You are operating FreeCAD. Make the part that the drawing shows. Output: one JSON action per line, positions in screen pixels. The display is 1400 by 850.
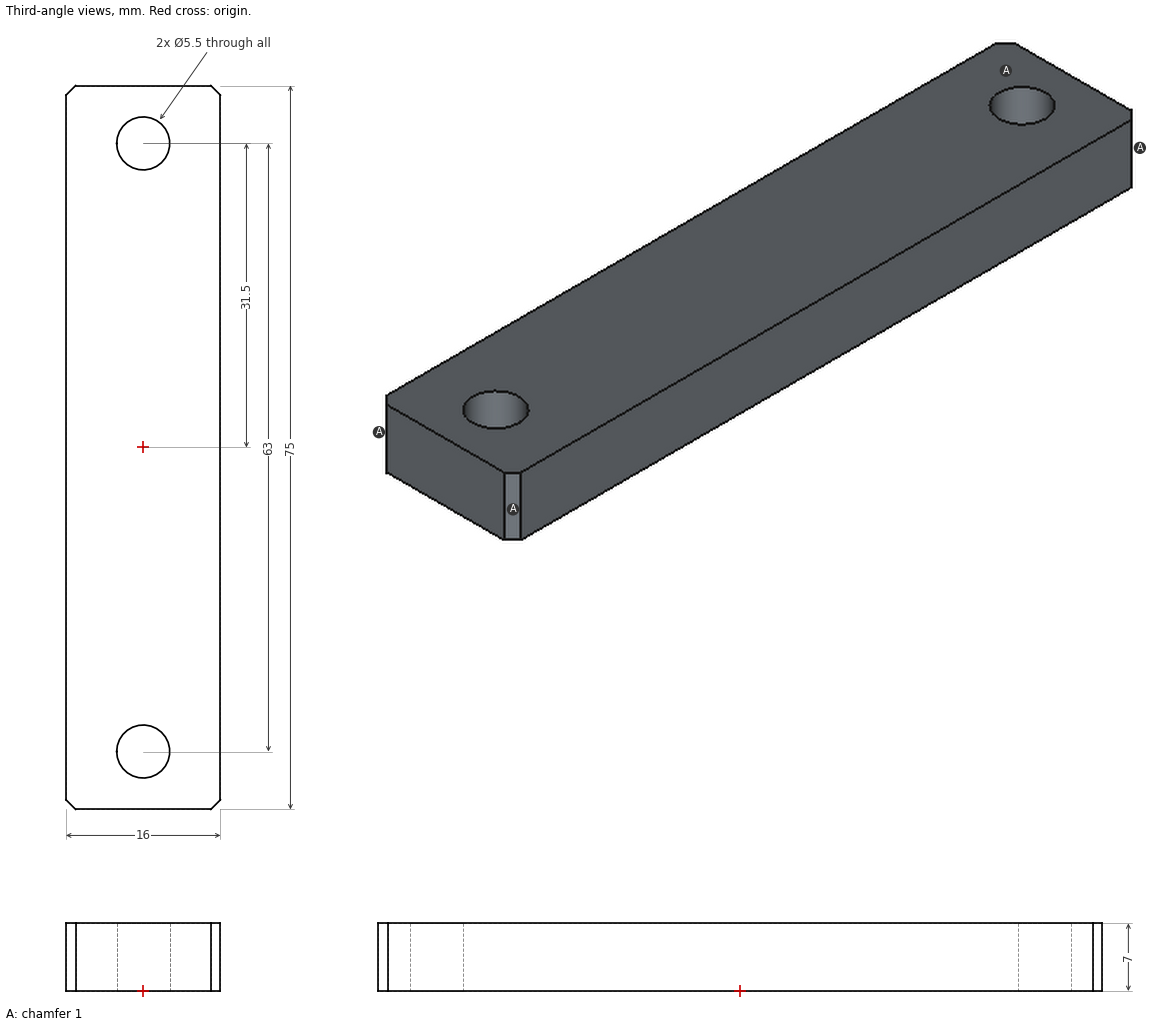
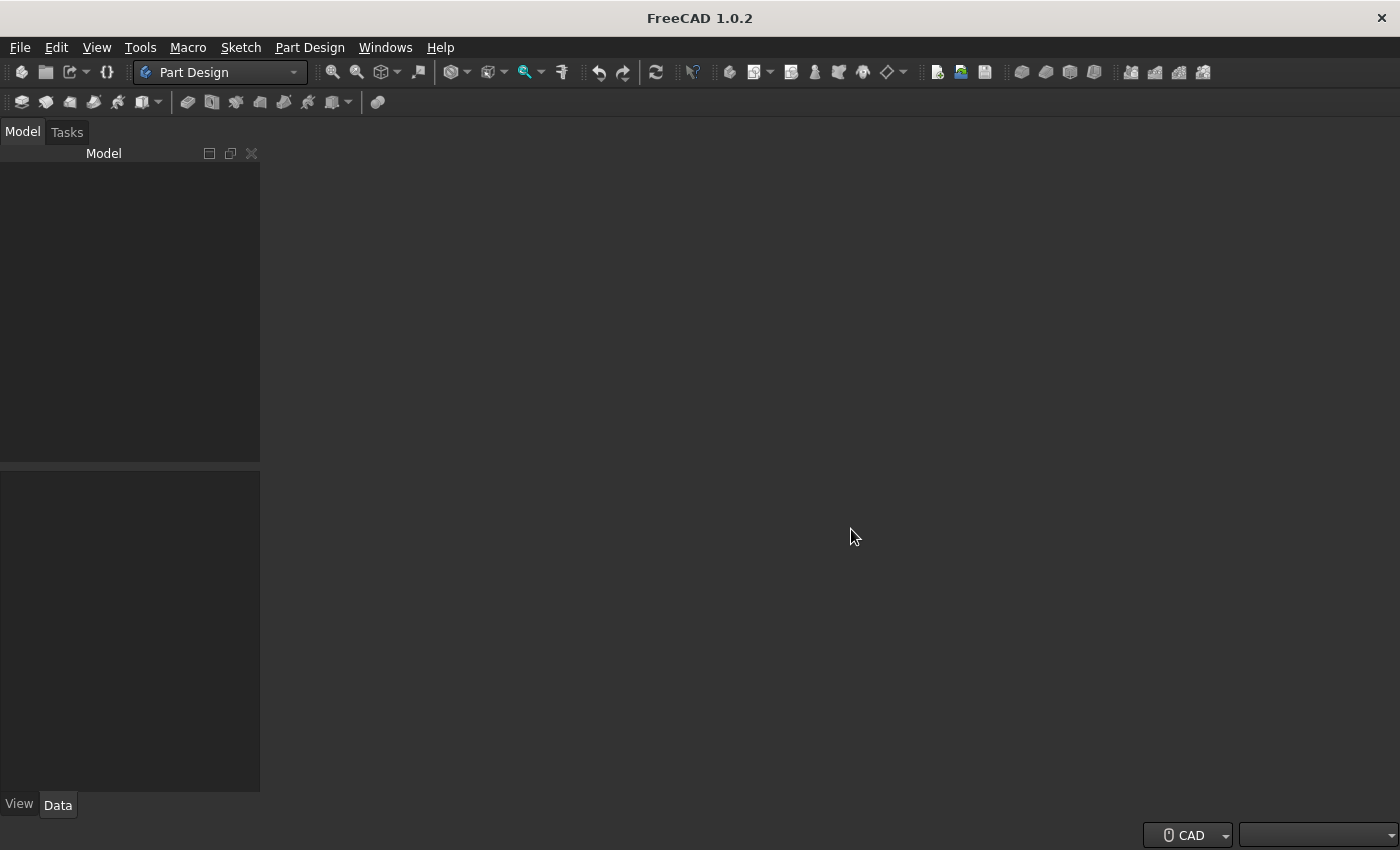
{"action": "left_click", "coordinate": [938, 72]}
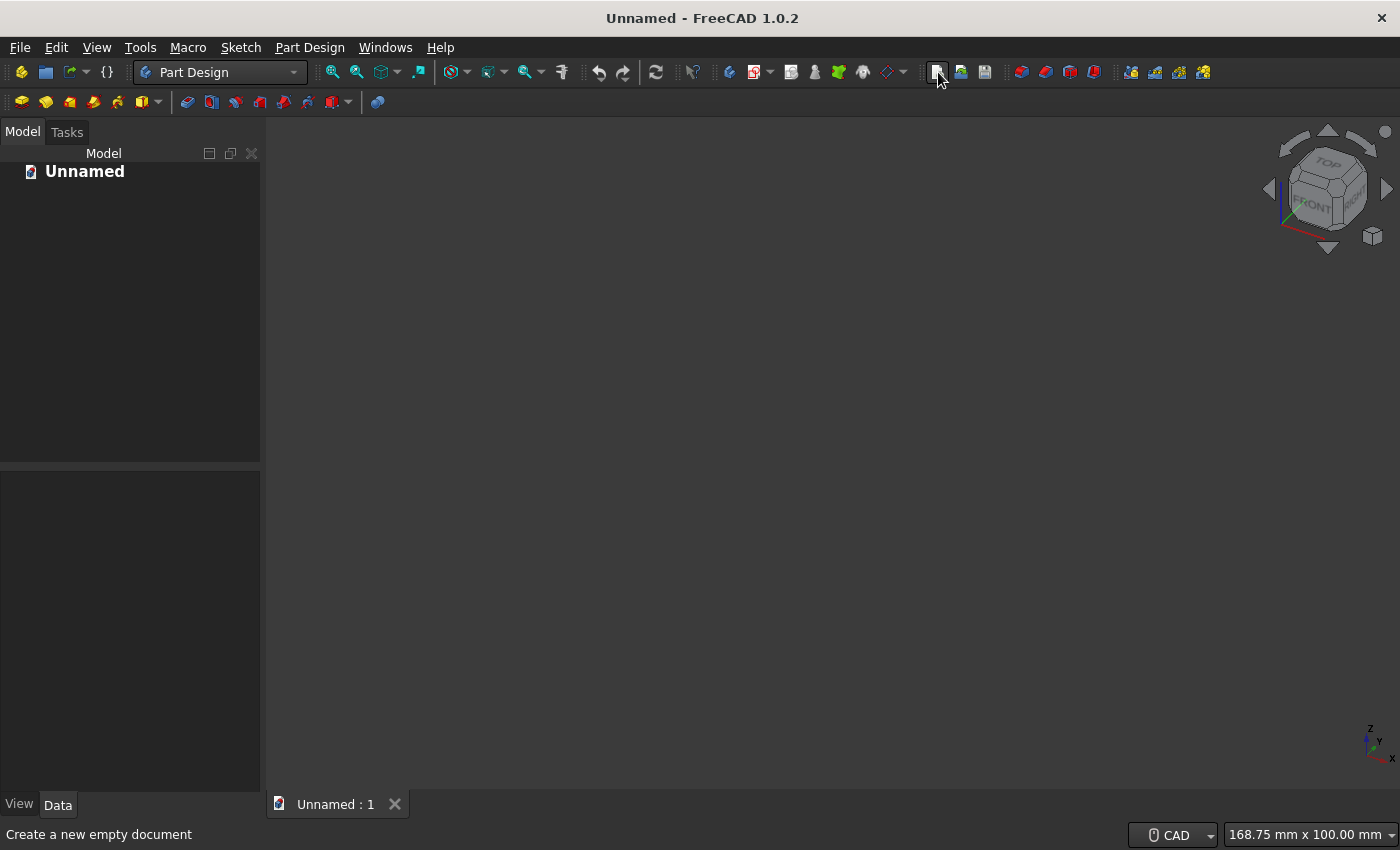
{"action": "left_click", "coordinate": [754, 72]}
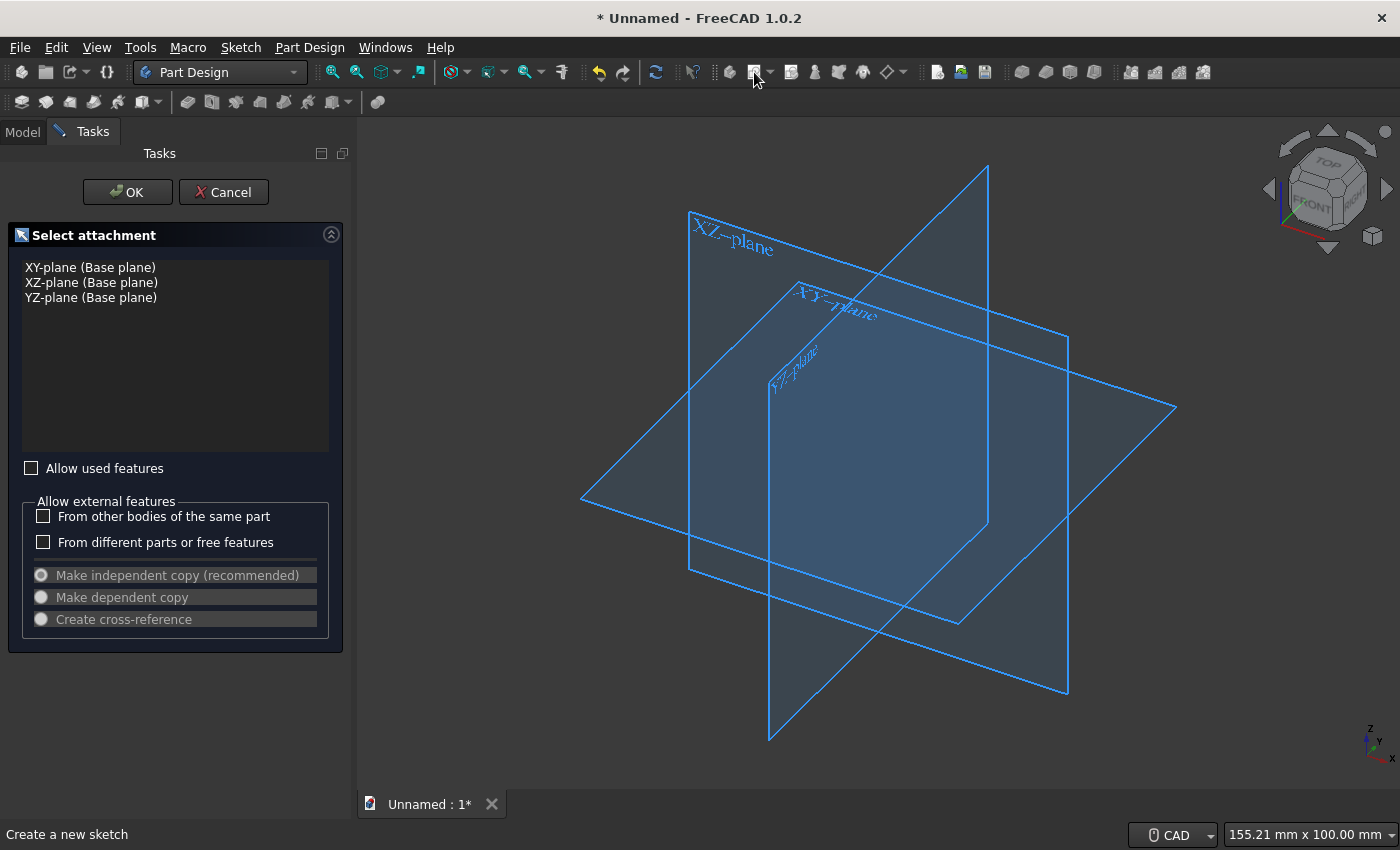
{"action": "left_click", "coordinate": [82, 268]}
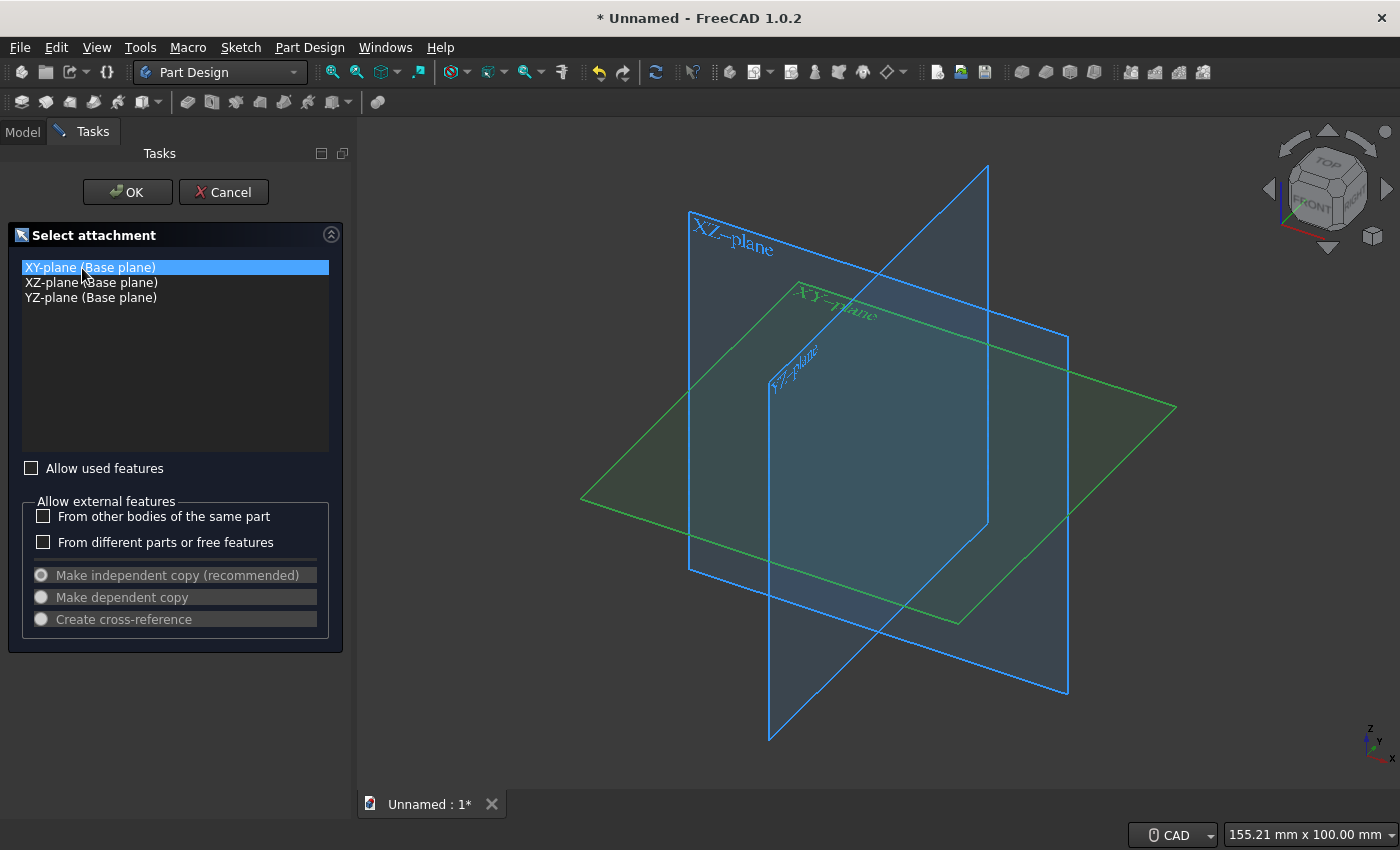
{"action": "left_click", "coordinate": [128, 192]}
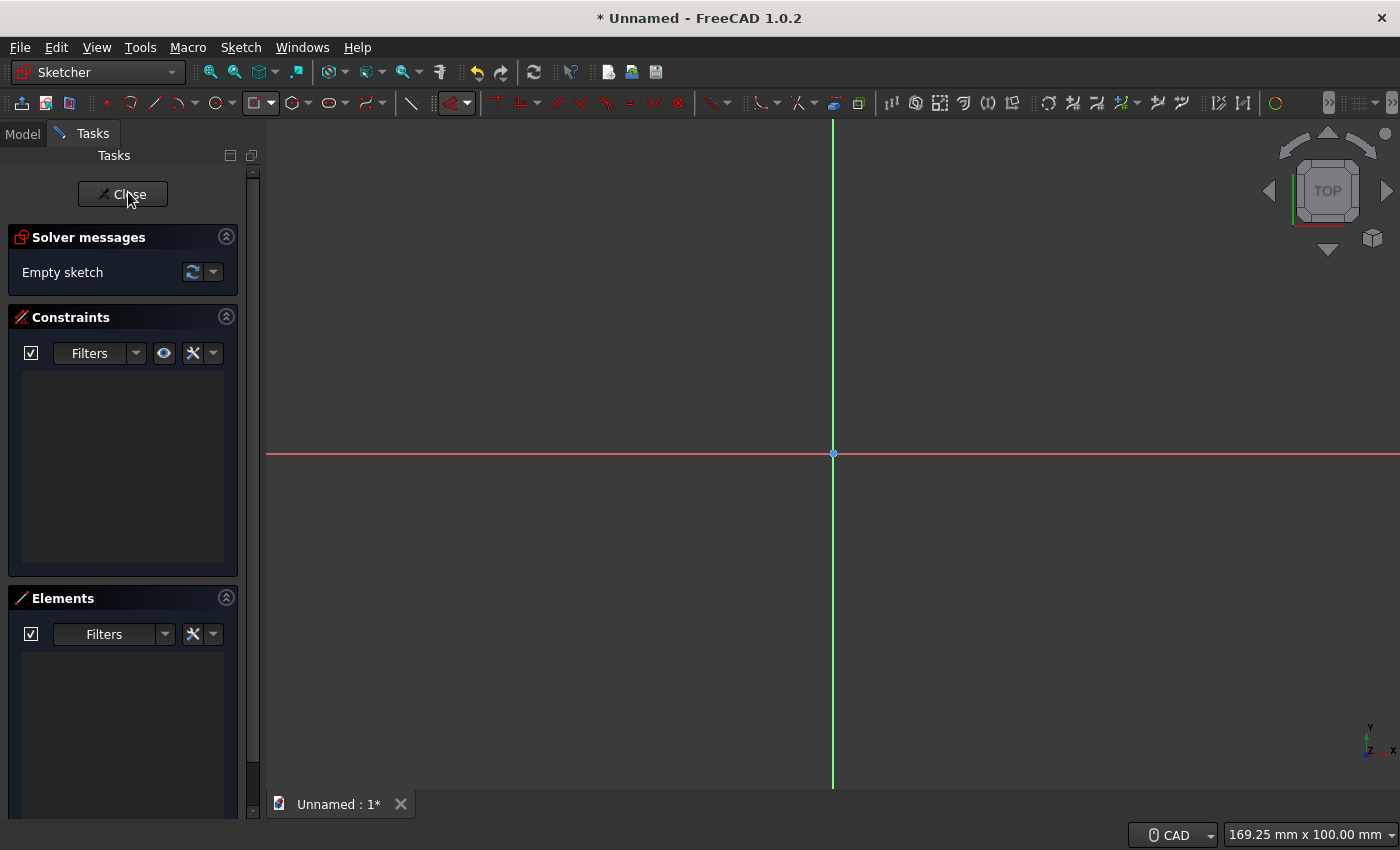
{"action": "left_click", "coordinate": [254, 104]}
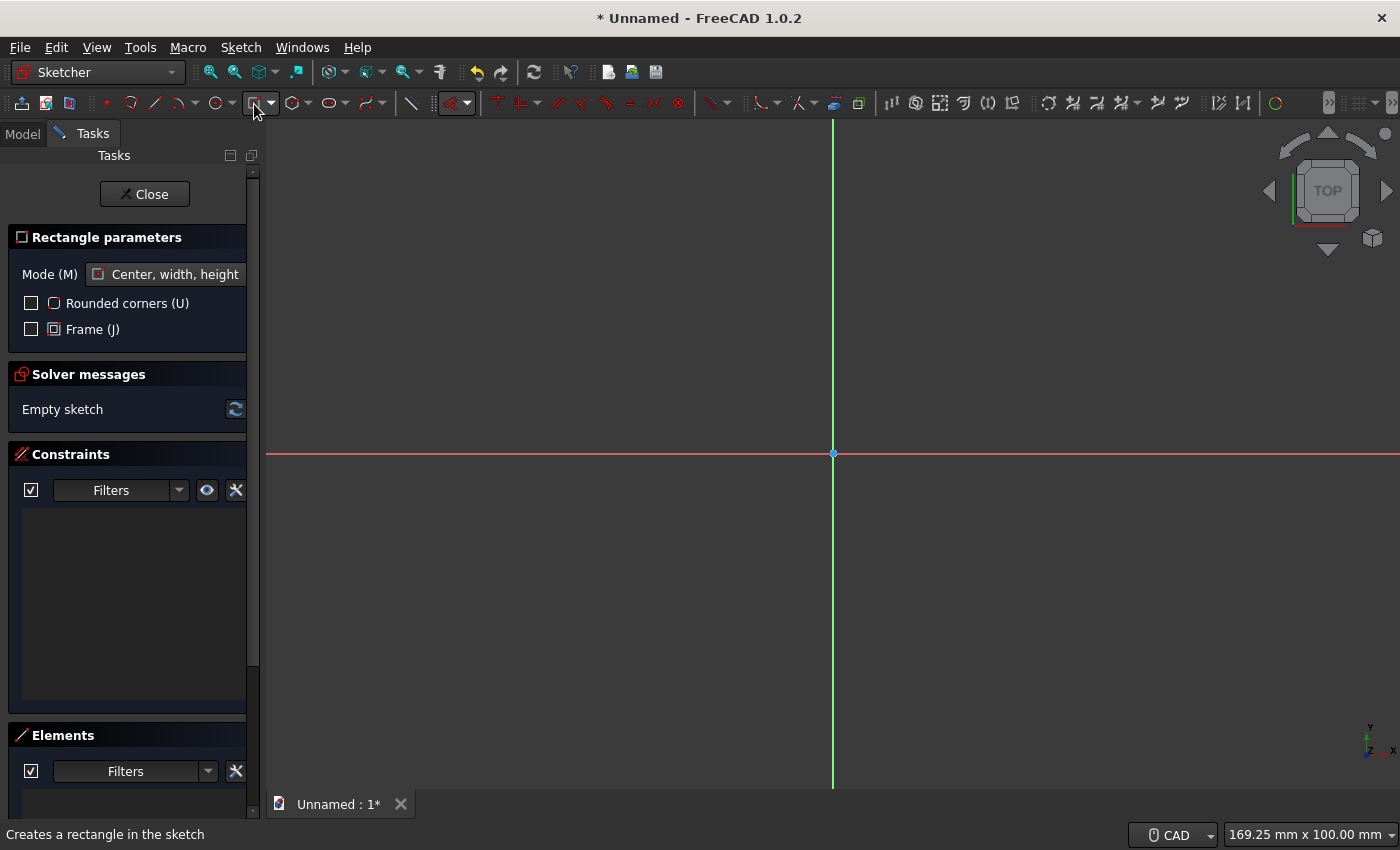
{"action": "left_click", "coordinate": [833, 454]}
{"action": "left_click", "coordinate": [887, 203]}
{"action": "key", "text": "Escape"}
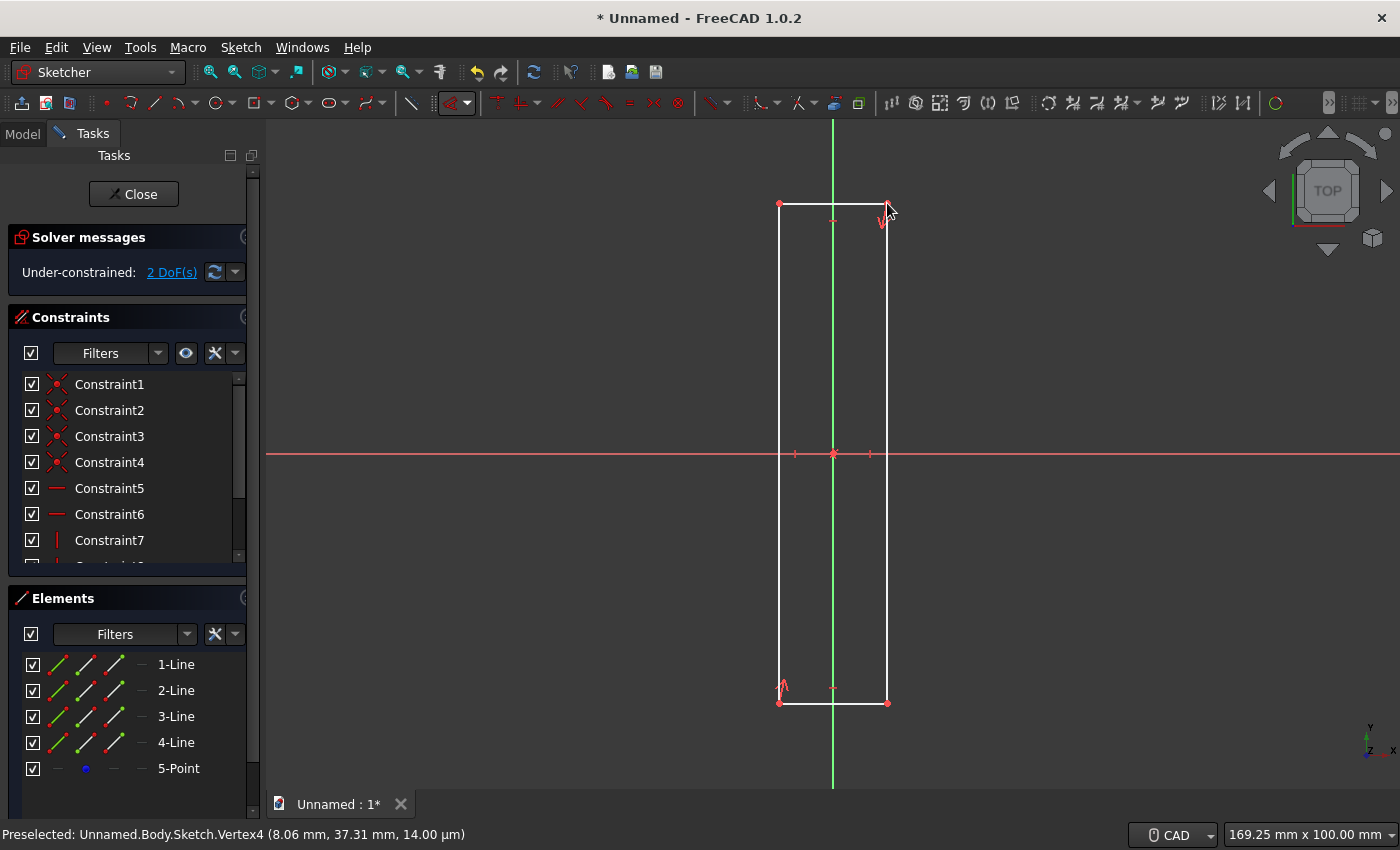
{"action": "left_click", "coordinate": [450, 104]}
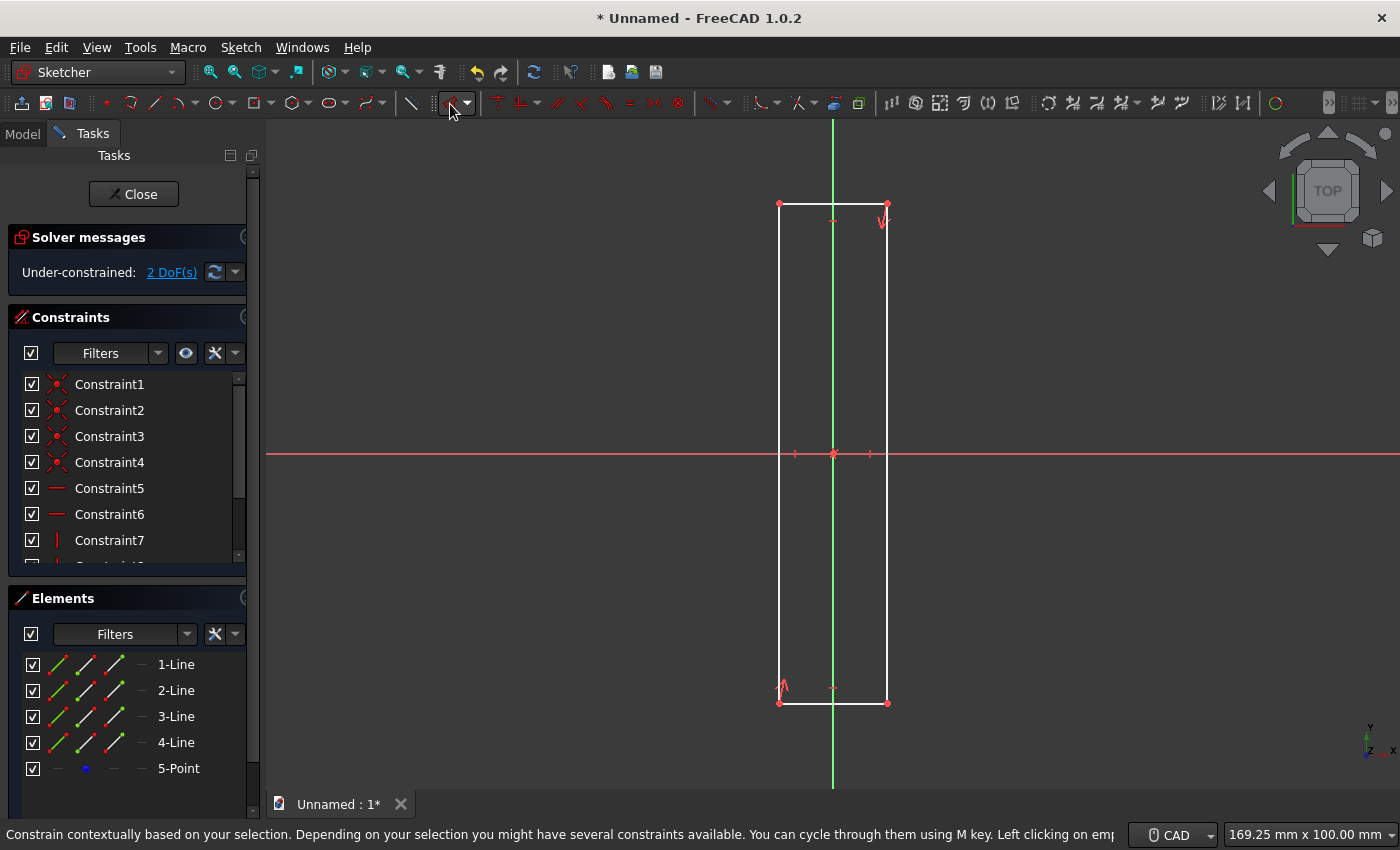
{"action": "left_click", "coordinate": [811, 704]}
{"action": "left_click", "coordinate": [808, 738]}